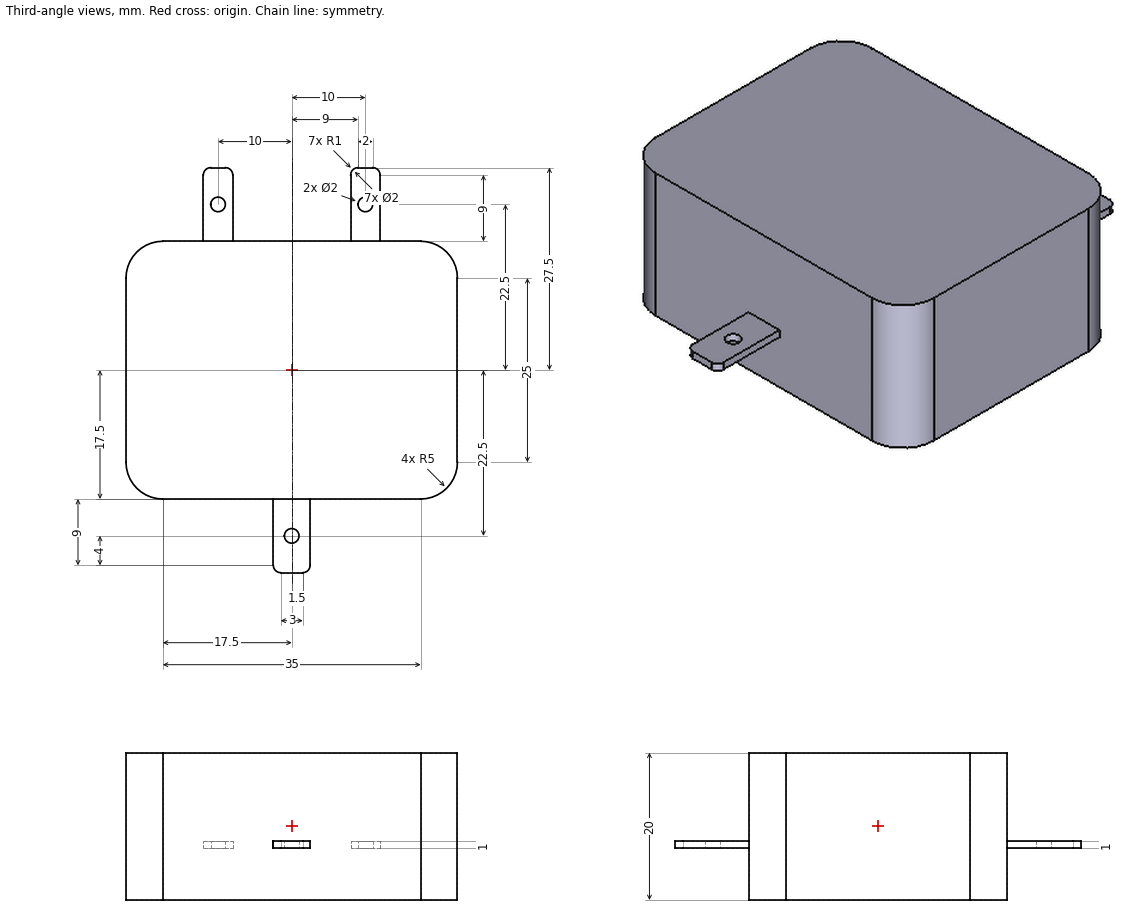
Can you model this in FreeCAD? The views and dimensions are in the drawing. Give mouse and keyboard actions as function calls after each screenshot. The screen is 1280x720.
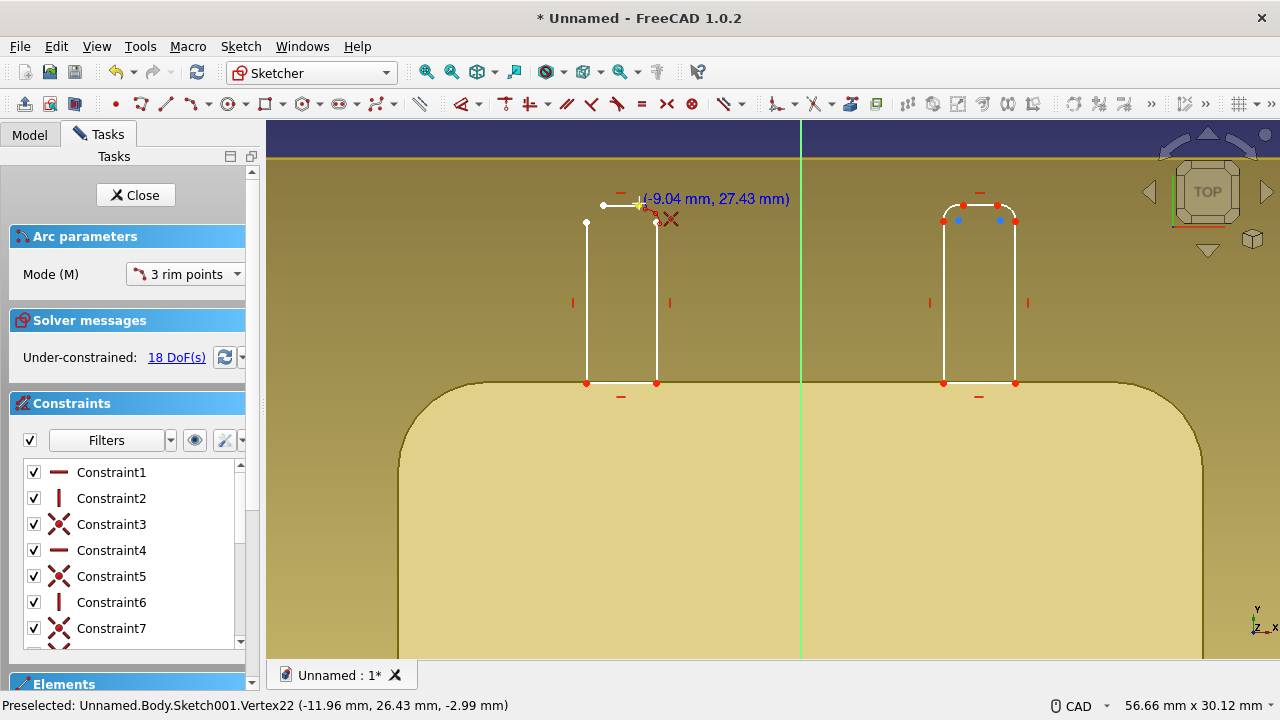
click(639, 206)
click(657, 222)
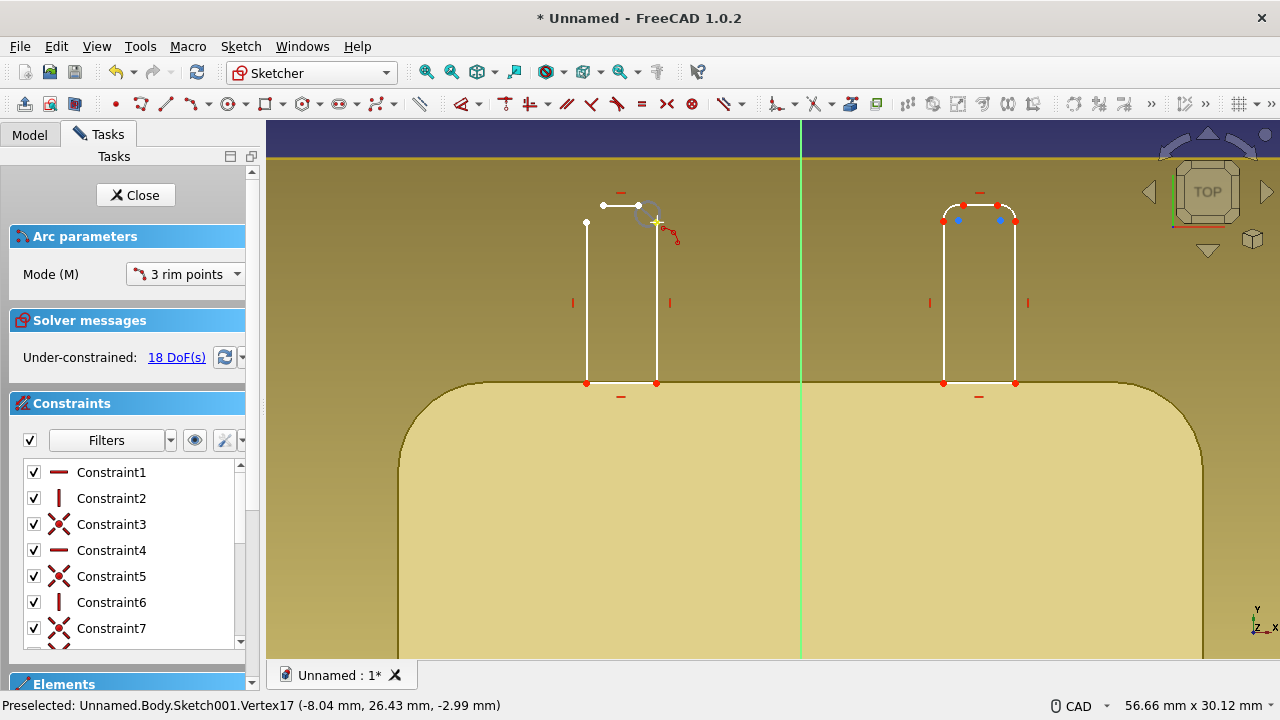
scroll(652, 208, up, 6)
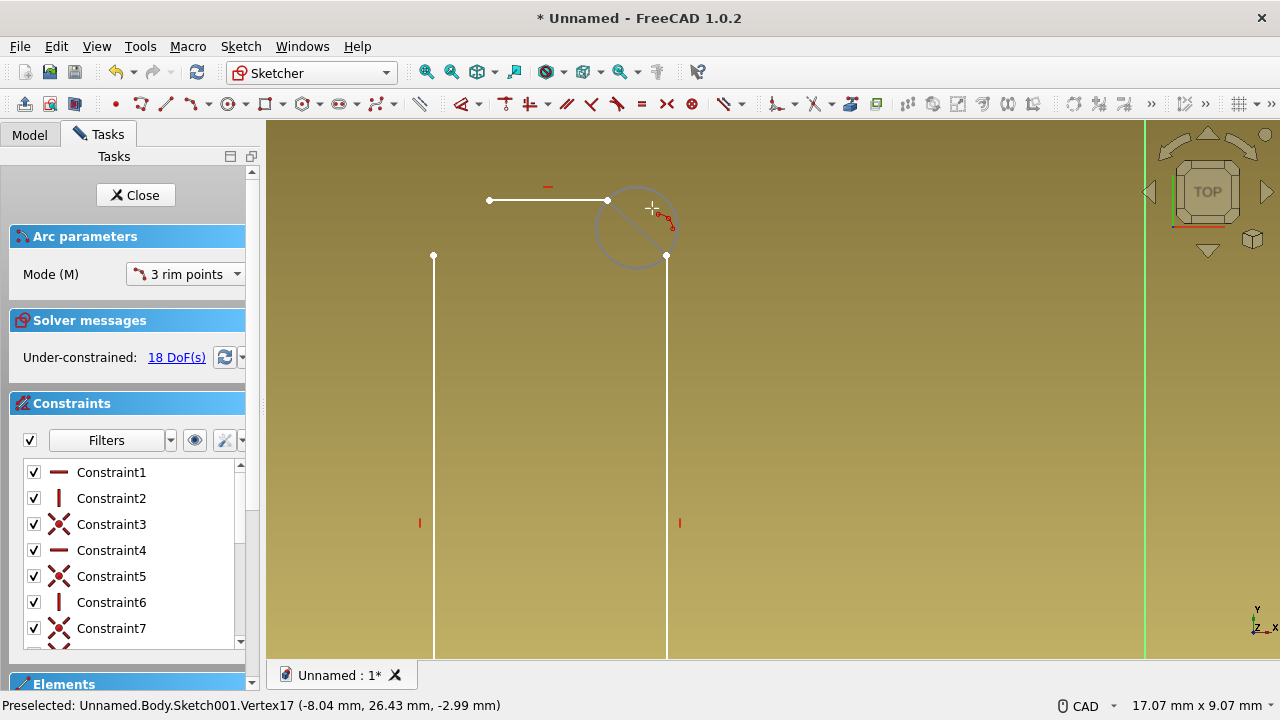
click(652, 209)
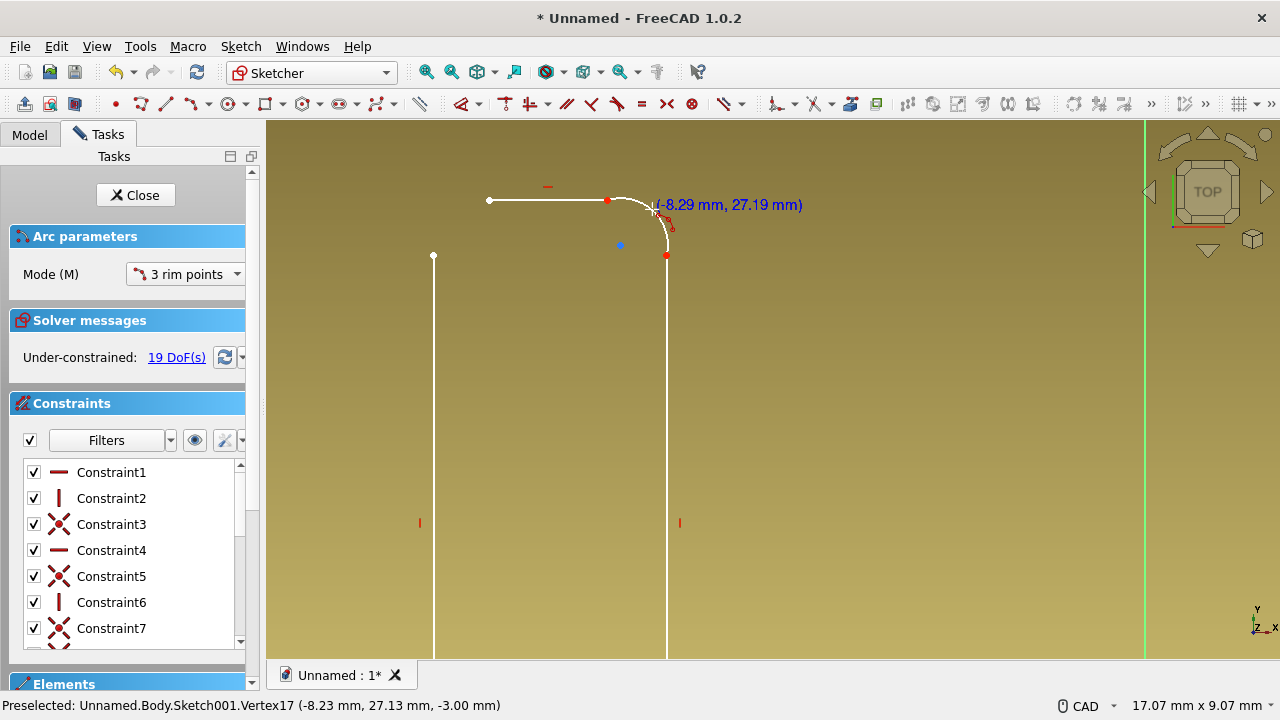
scroll(650, 211, down, 11)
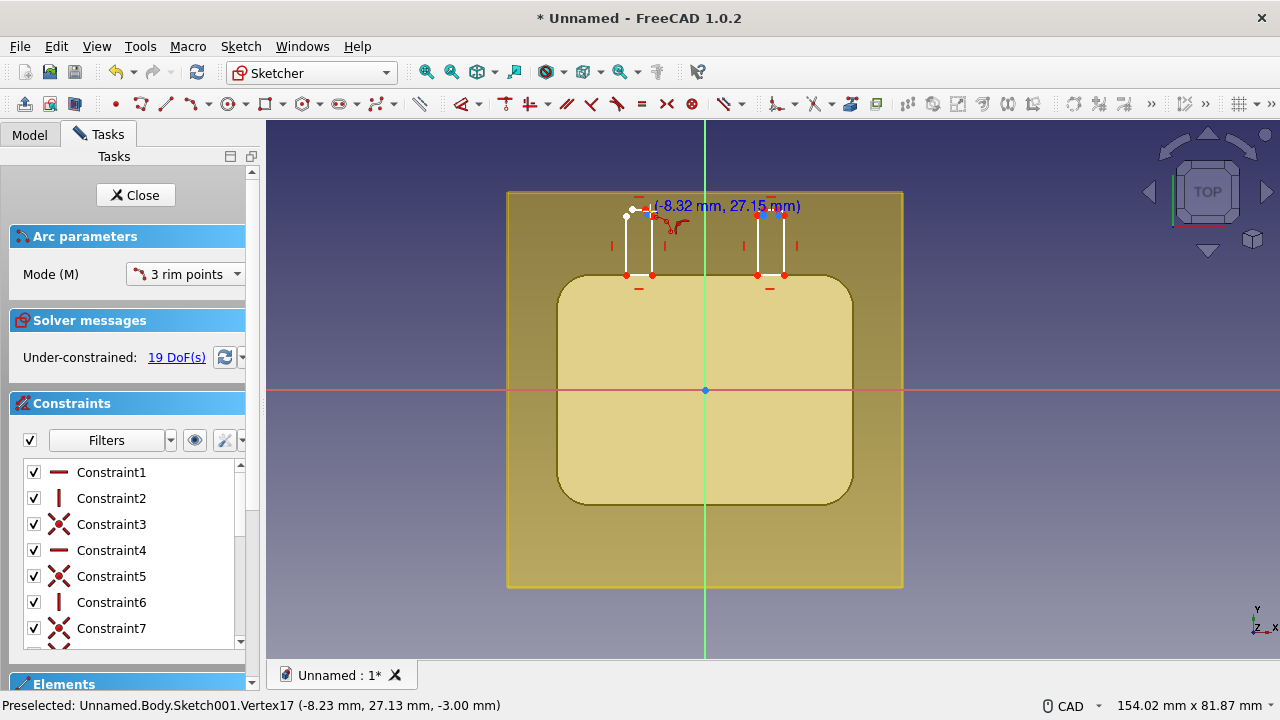
scroll(626, 216, up, 3)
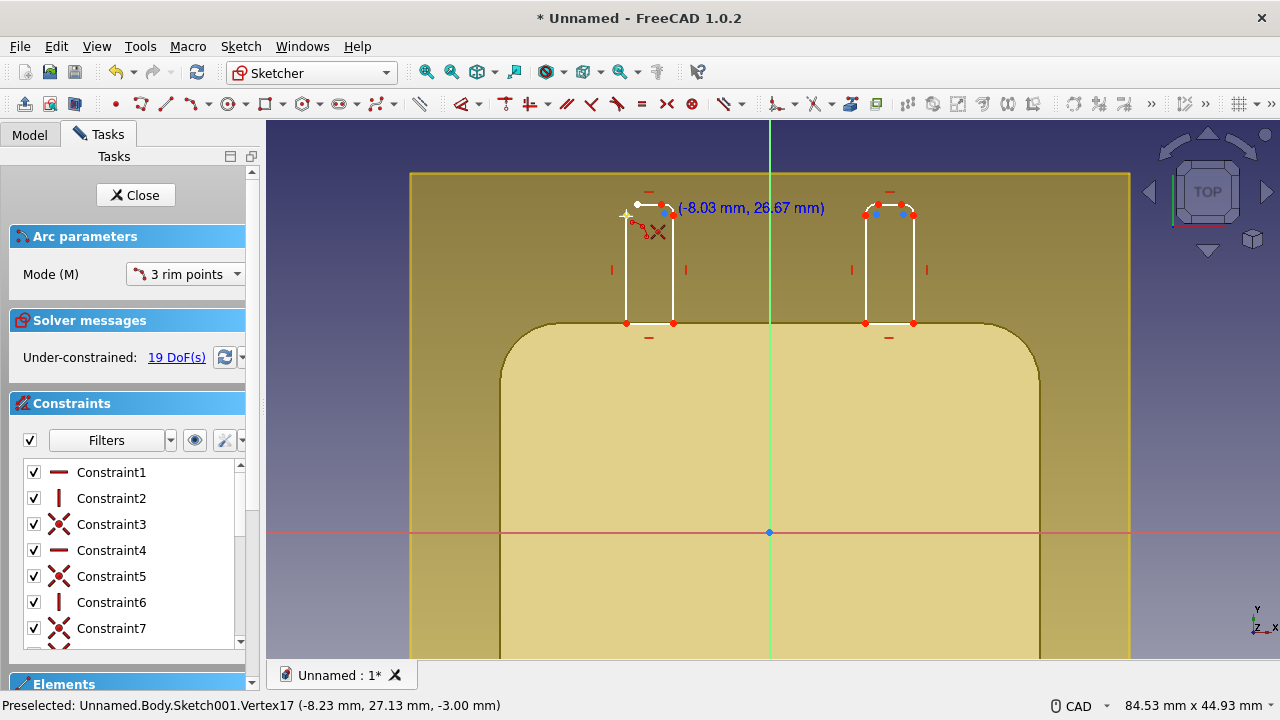
click(626, 216)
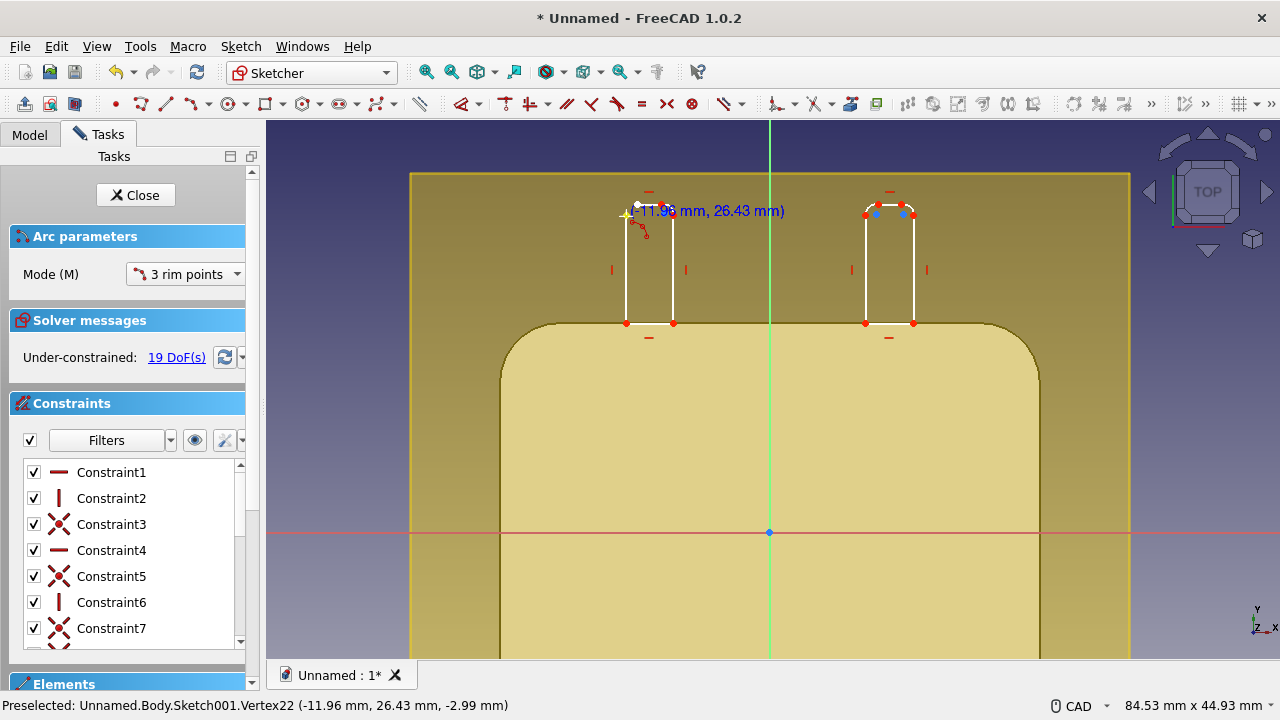
scroll(638, 203, up, 2)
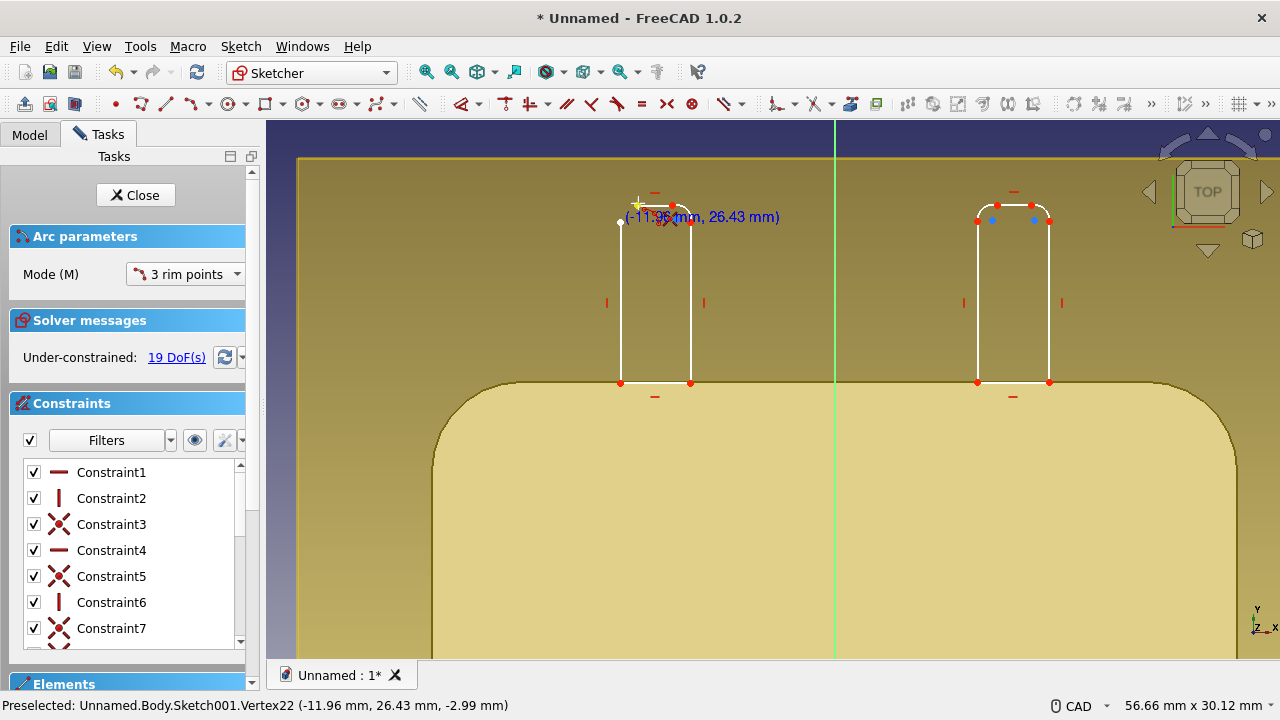
click(637, 206)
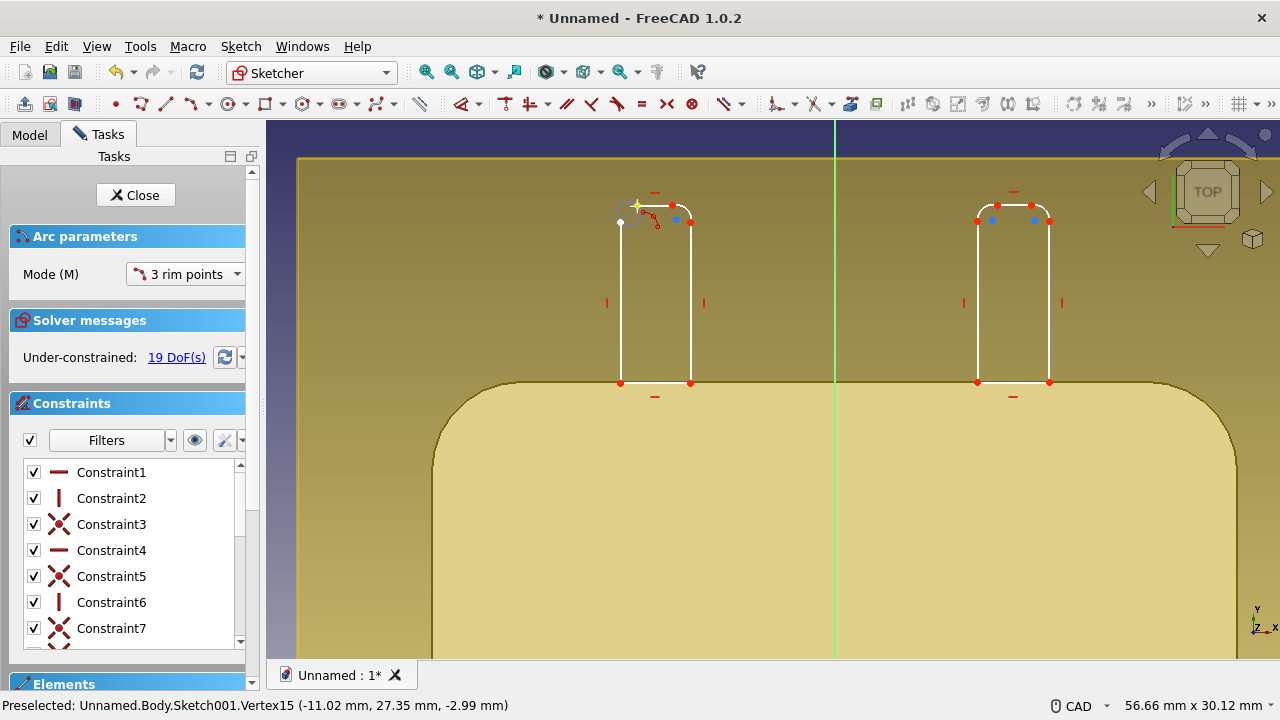
scroll(625, 208, up, 6)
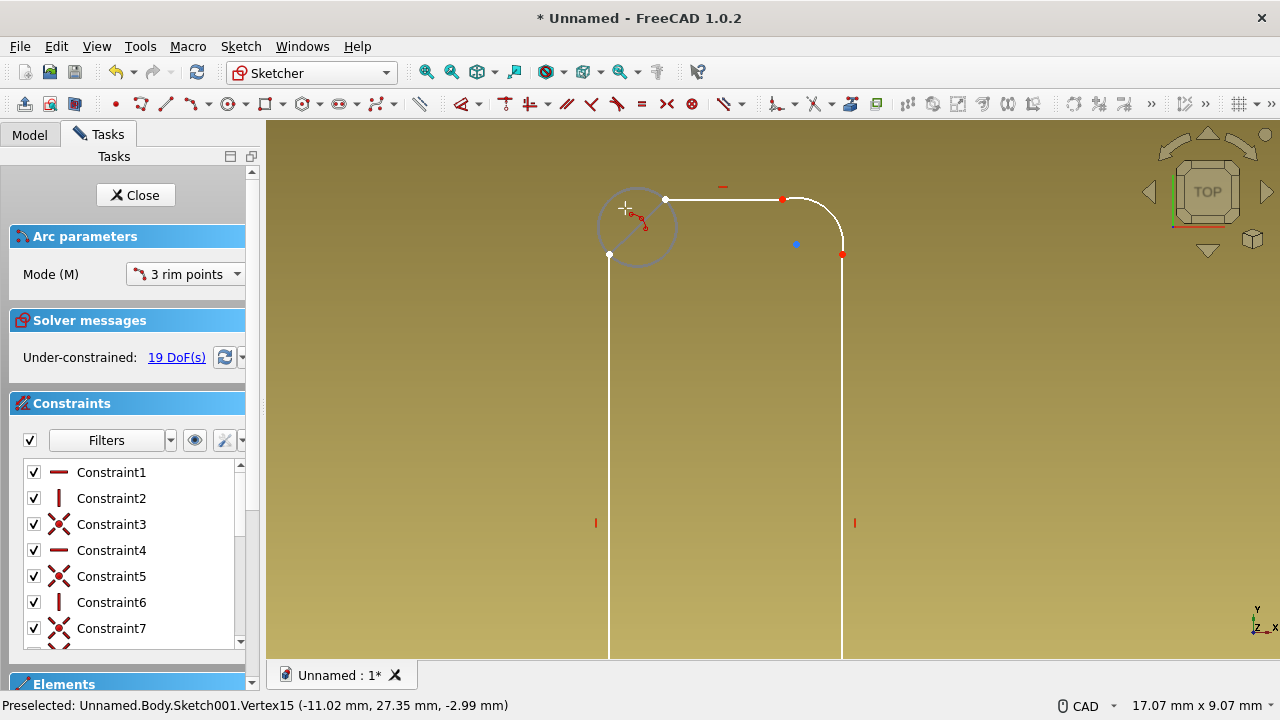
click(624, 208)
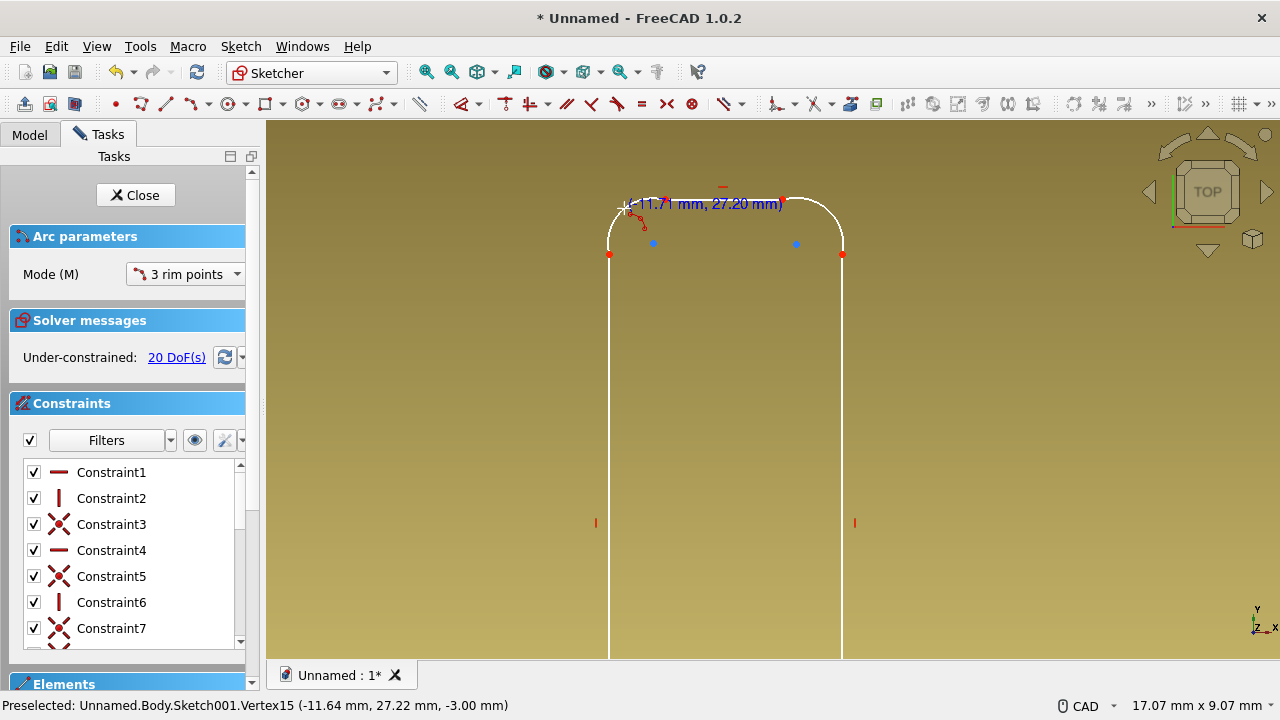
key(g)
key(l)